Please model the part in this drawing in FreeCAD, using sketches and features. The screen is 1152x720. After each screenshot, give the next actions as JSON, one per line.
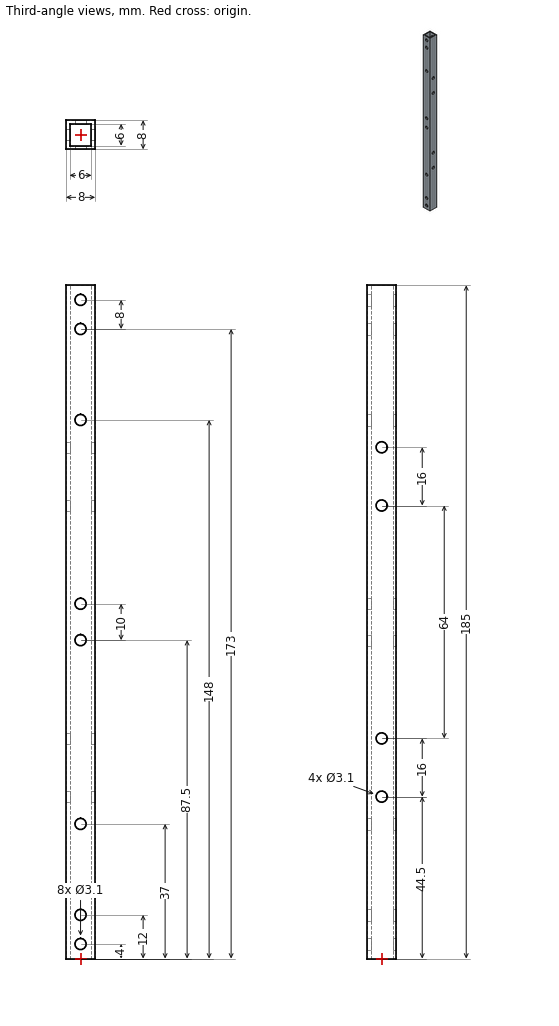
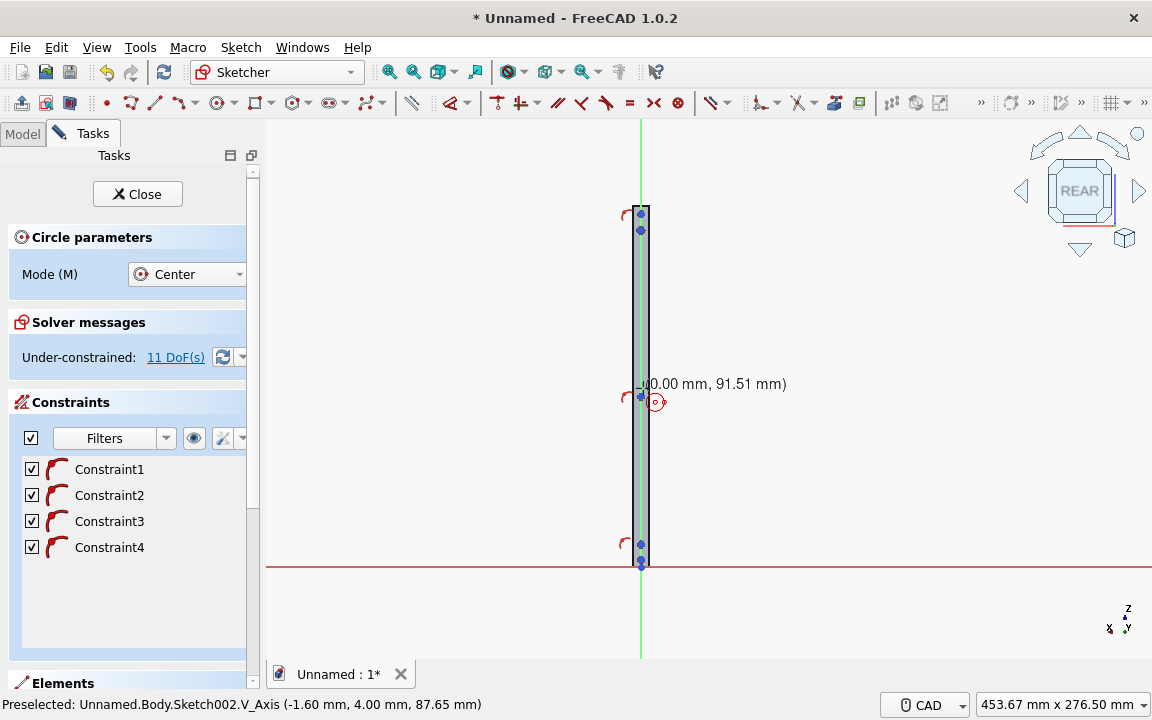
{"action": "left_click", "coordinate": [641, 377]}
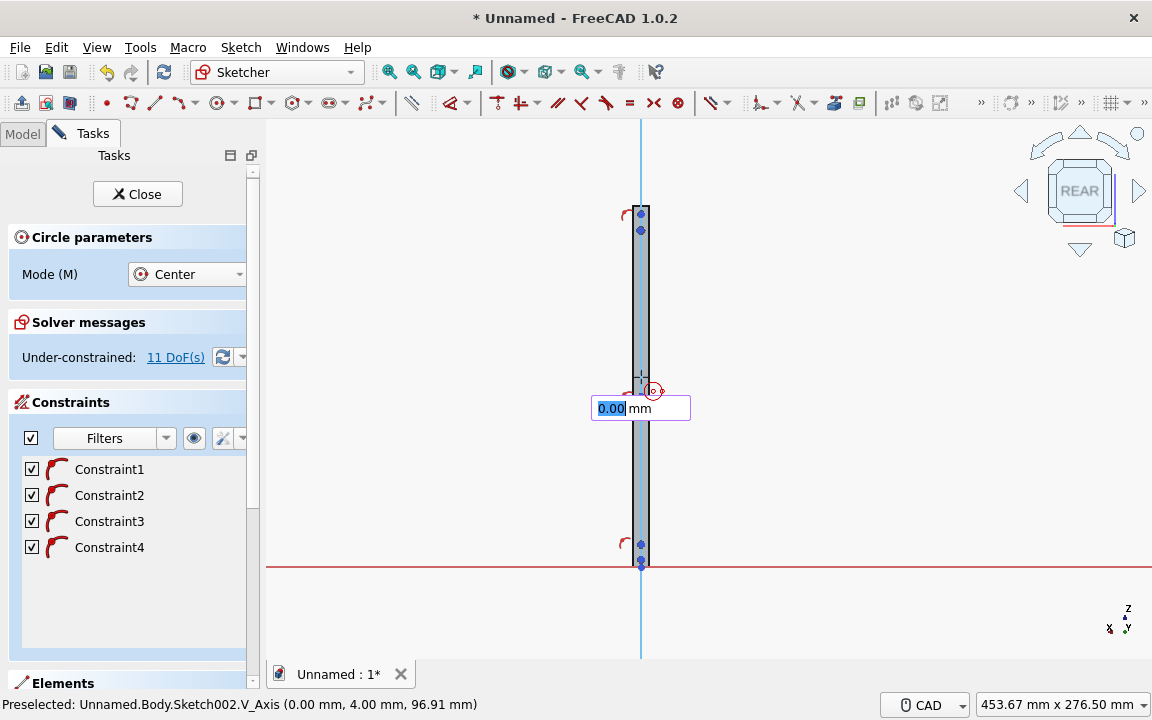
{"action": "scroll", "coordinate": [644, 376], "scroll_direction": "up", "scroll_amount": 9}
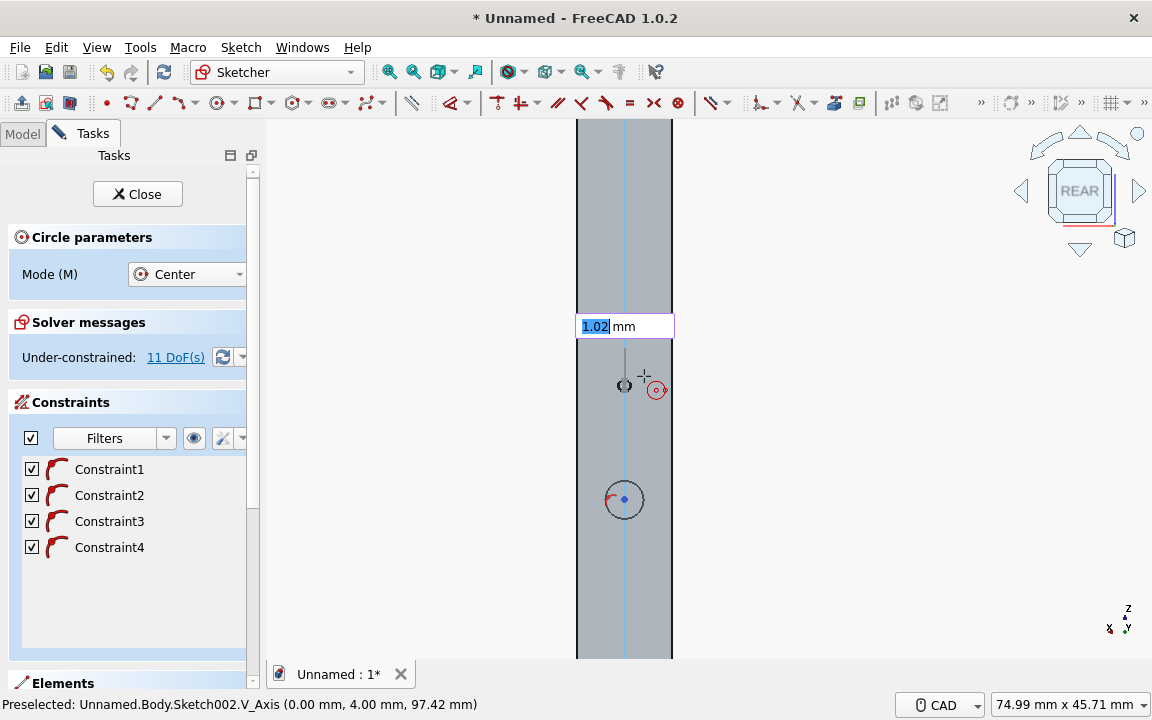
{"action": "left_click", "coordinate": [642, 372]}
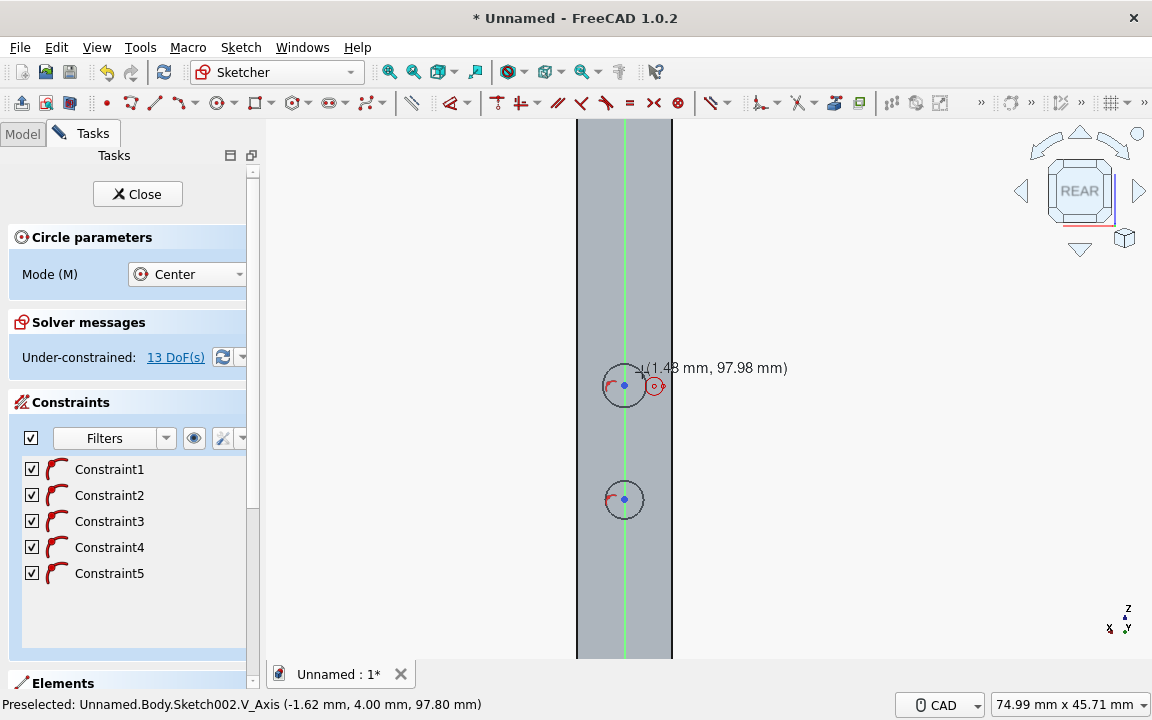
{"action": "scroll", "coordinate": [644, 376], "scroll_direction": "down", "scroll_amount": 9}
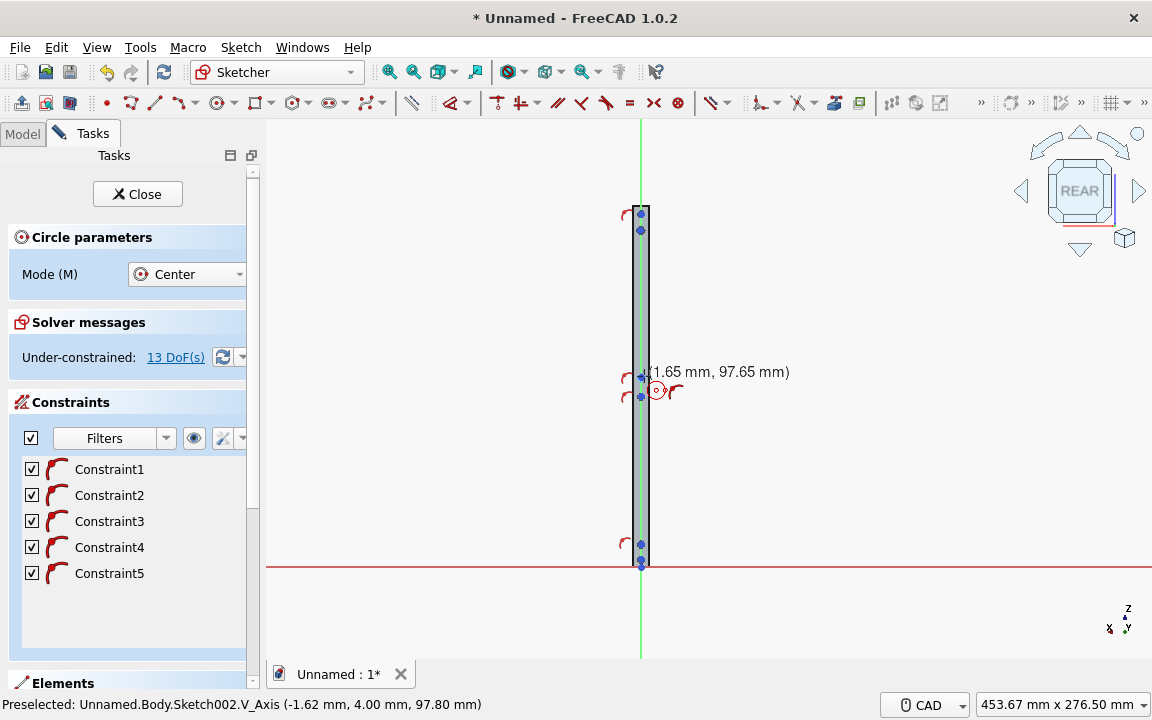
{"action": "scroll", "coordinate": [641, 278], "scroll_direction": "up", "scroll_amount": 11}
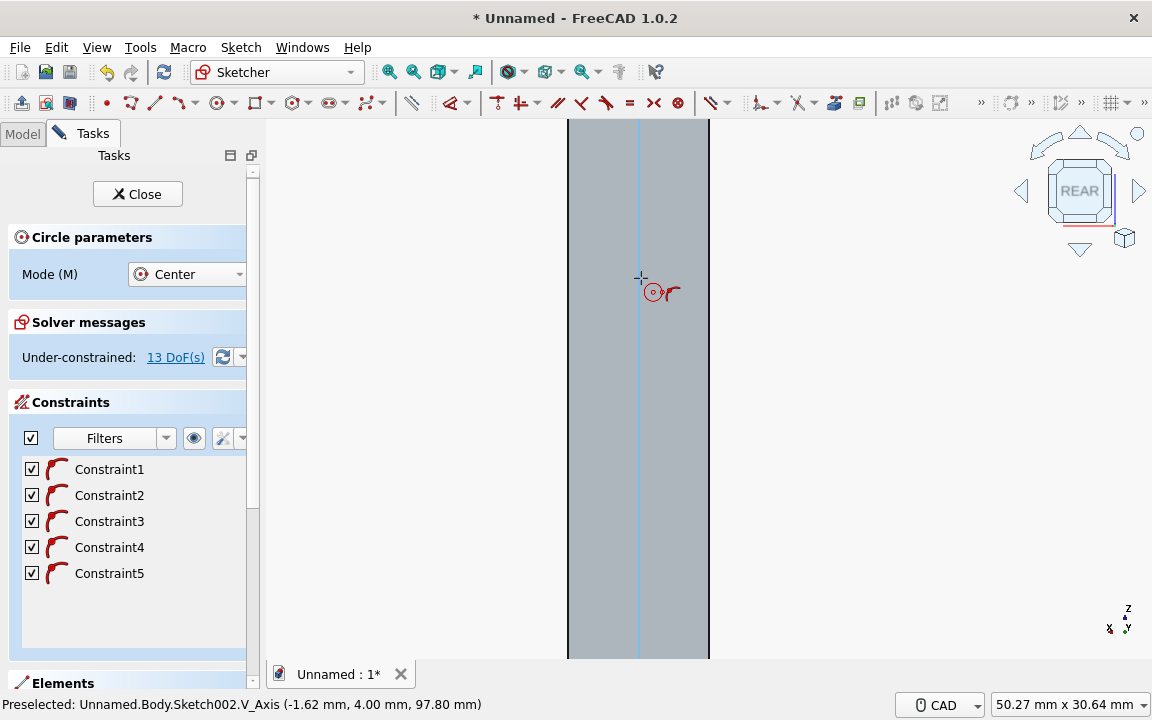
{"action": "scroll", "coordinate": [641, 278], "scroll_direction": "down", "scroll_amount": 11}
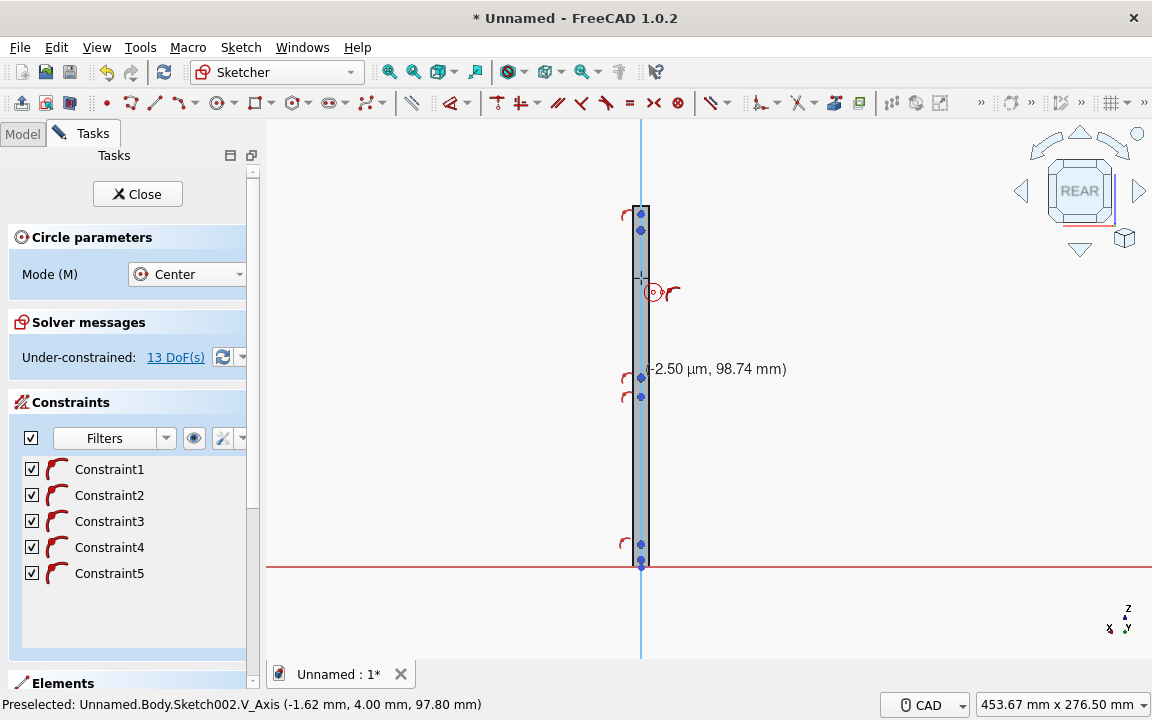
{"action": "left_click", "coordinate": [641, 278]}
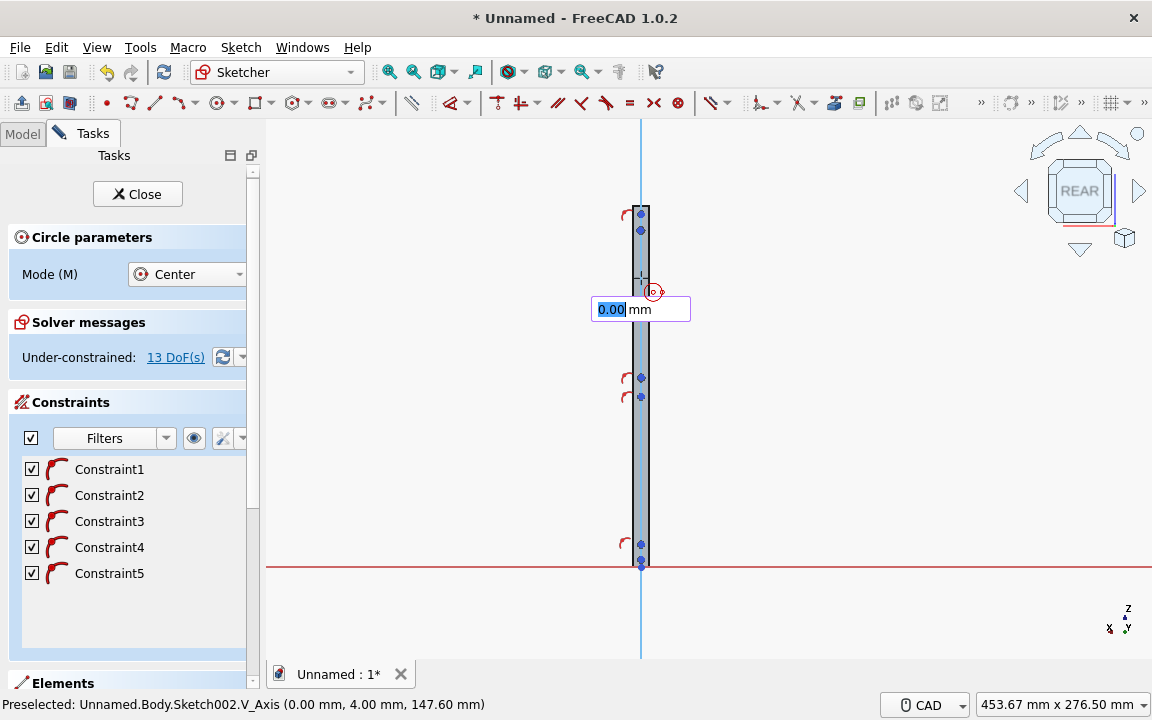
{"action": "scroll", "coordinate": [644, 277], "scroll_direction": "up", "scroll_amount": 9}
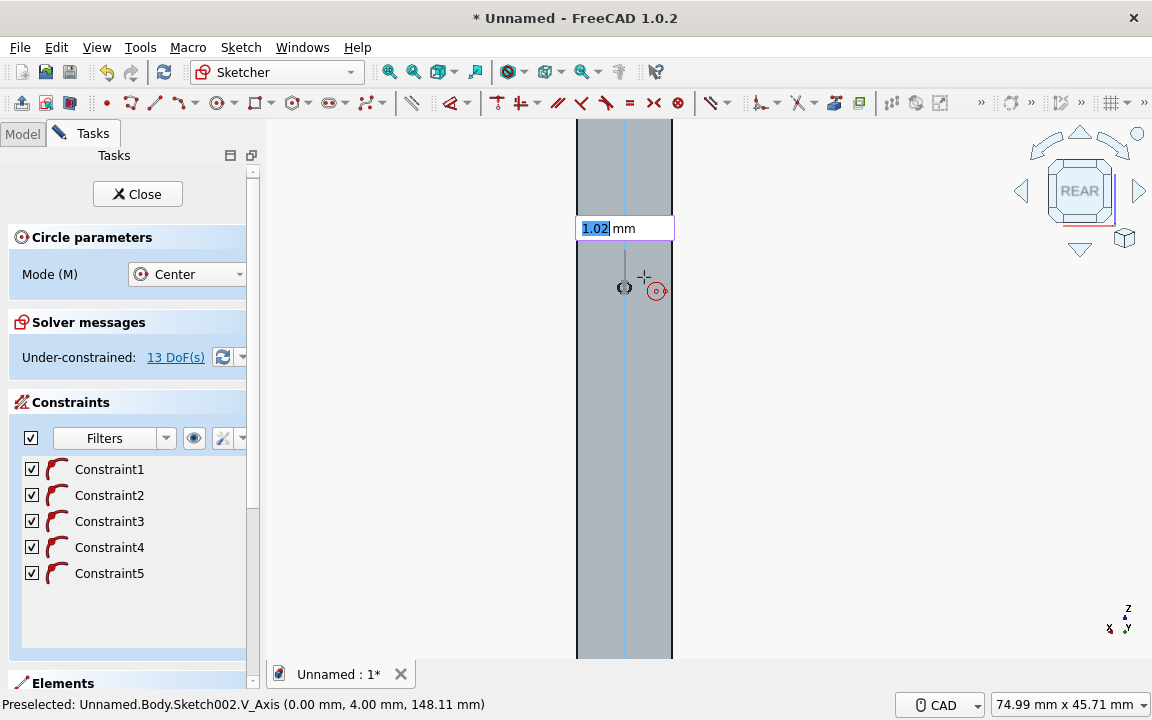
{"action": "left_click", "coordinate": [642, 277]}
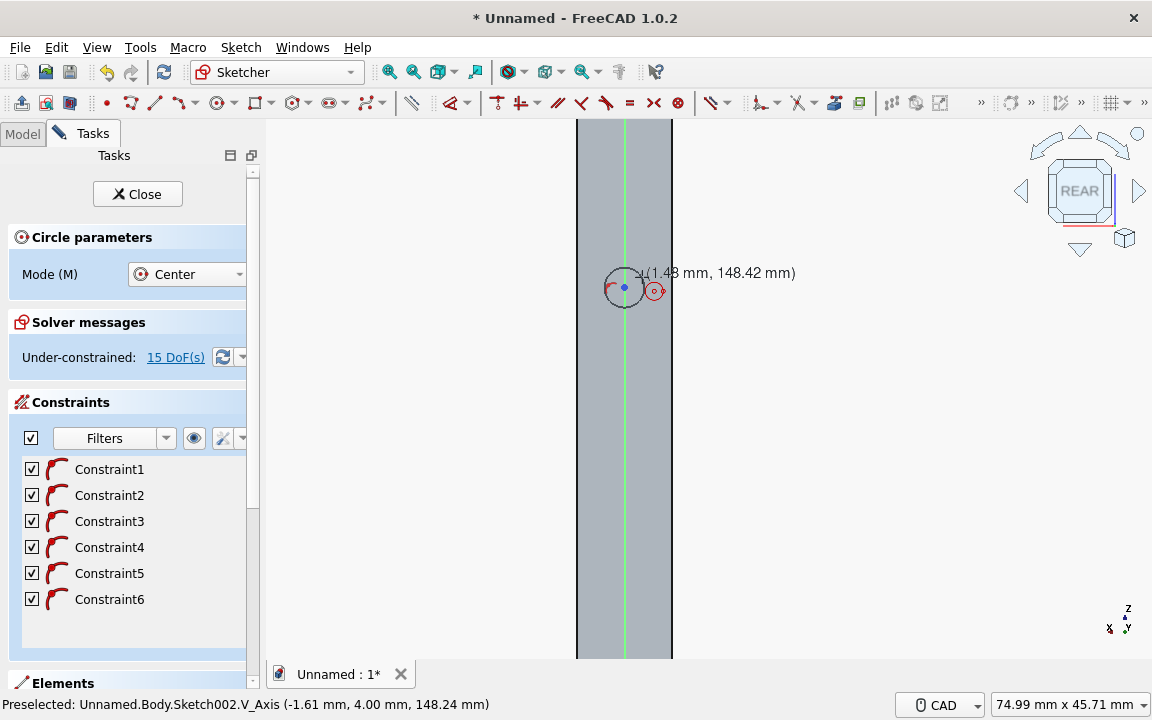
{"action": "scroll", "coordinate": [644, 277], "scroll_direction": "down", "scroll_amount": 9}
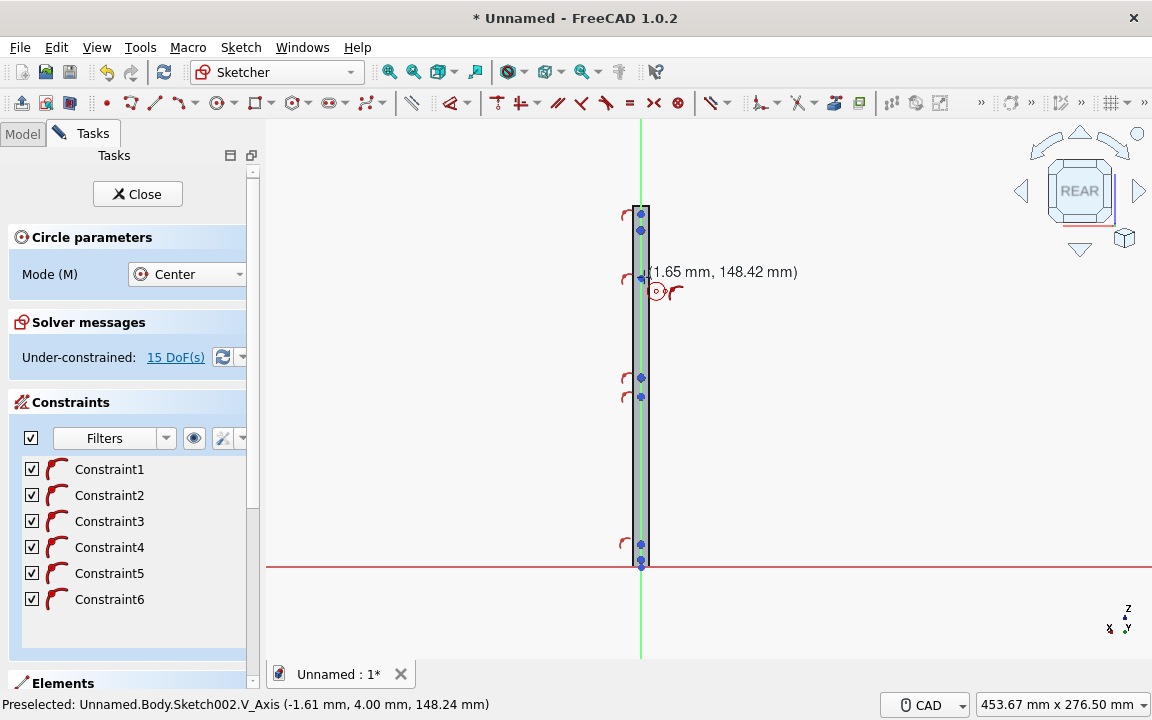
{"action": "scroll", "coordinate": [641, 495], "scroll_direction": "up", "scroll_amount": 11}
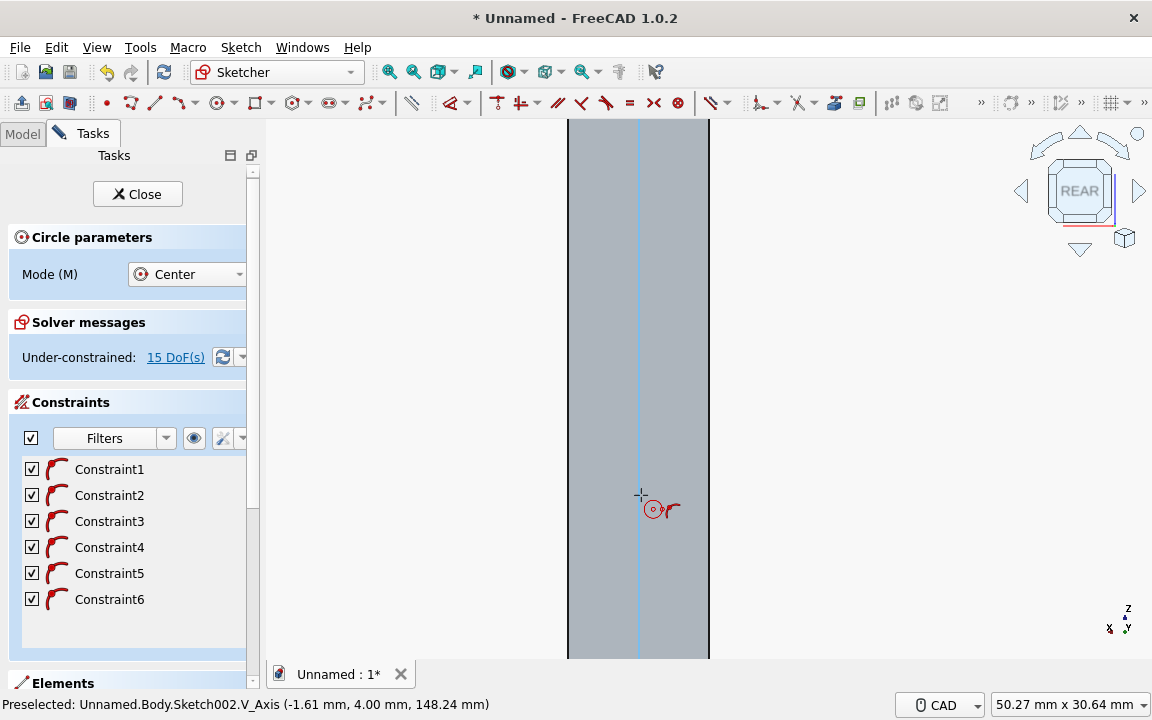
{"action": "scroll", "coordinate": [641, 496], "scroll_direction": "down", "scroll_amount": 11}